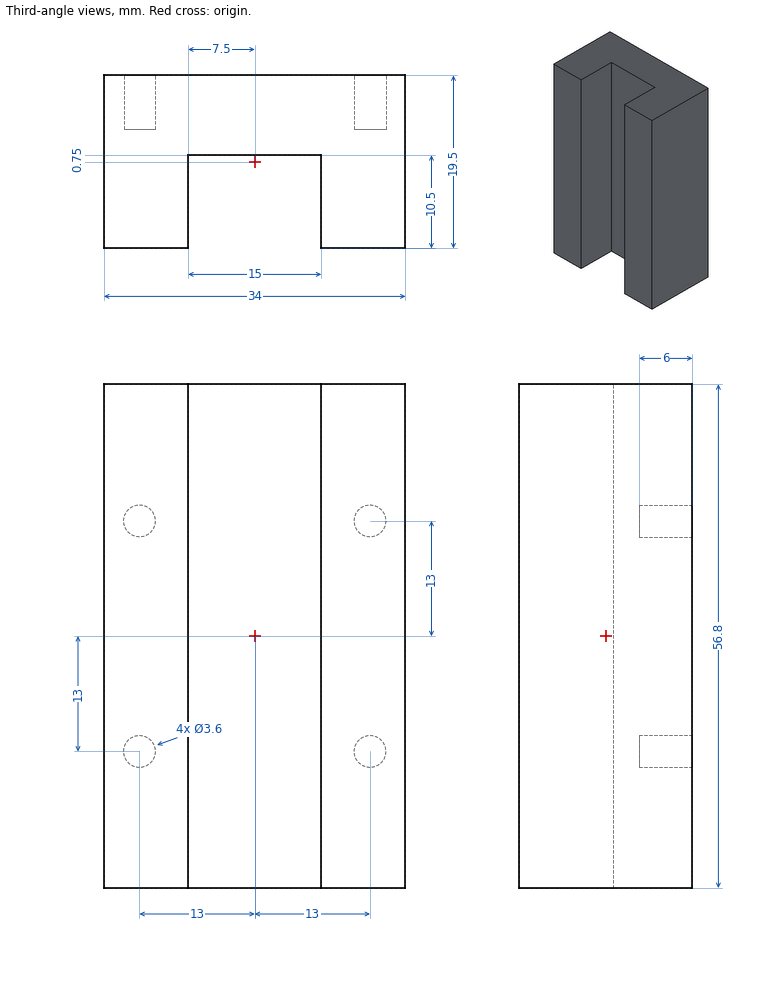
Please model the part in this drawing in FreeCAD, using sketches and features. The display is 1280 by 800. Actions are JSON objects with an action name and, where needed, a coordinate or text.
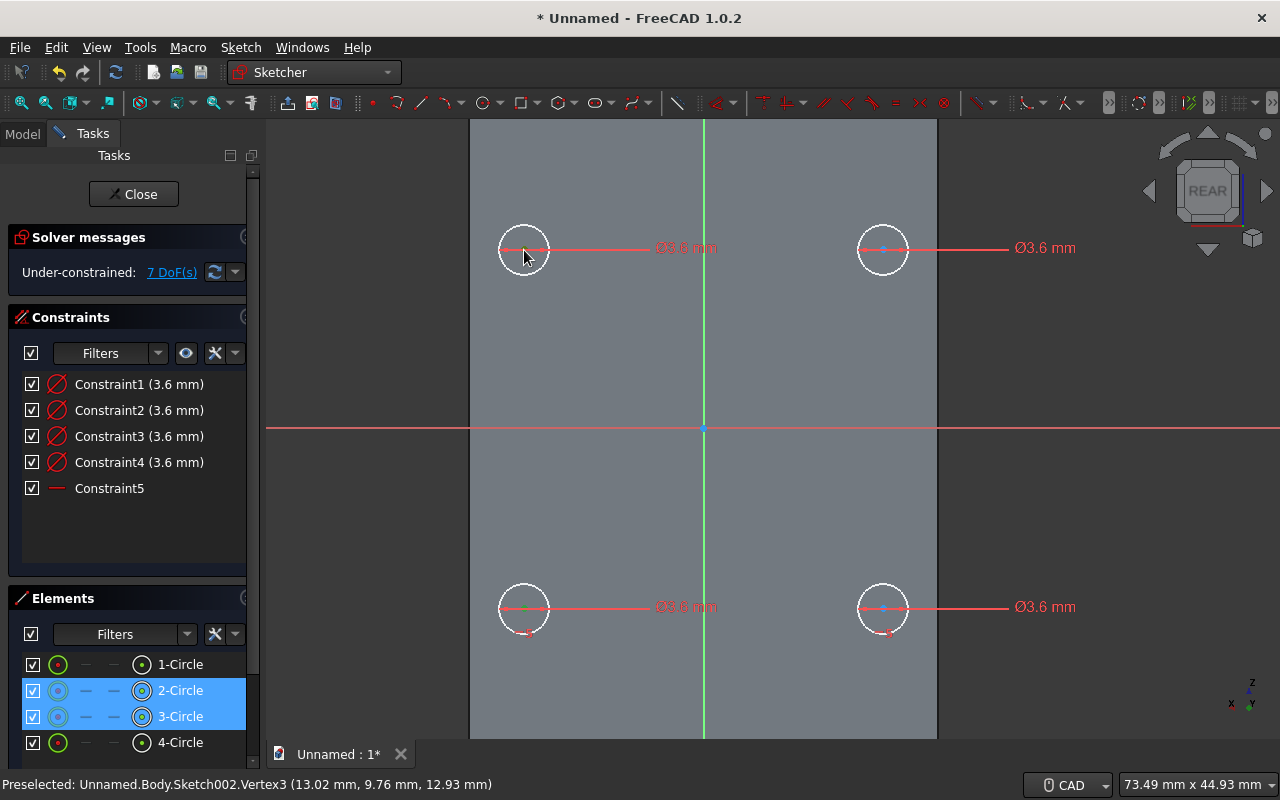
{"action": "key", "text": "v"}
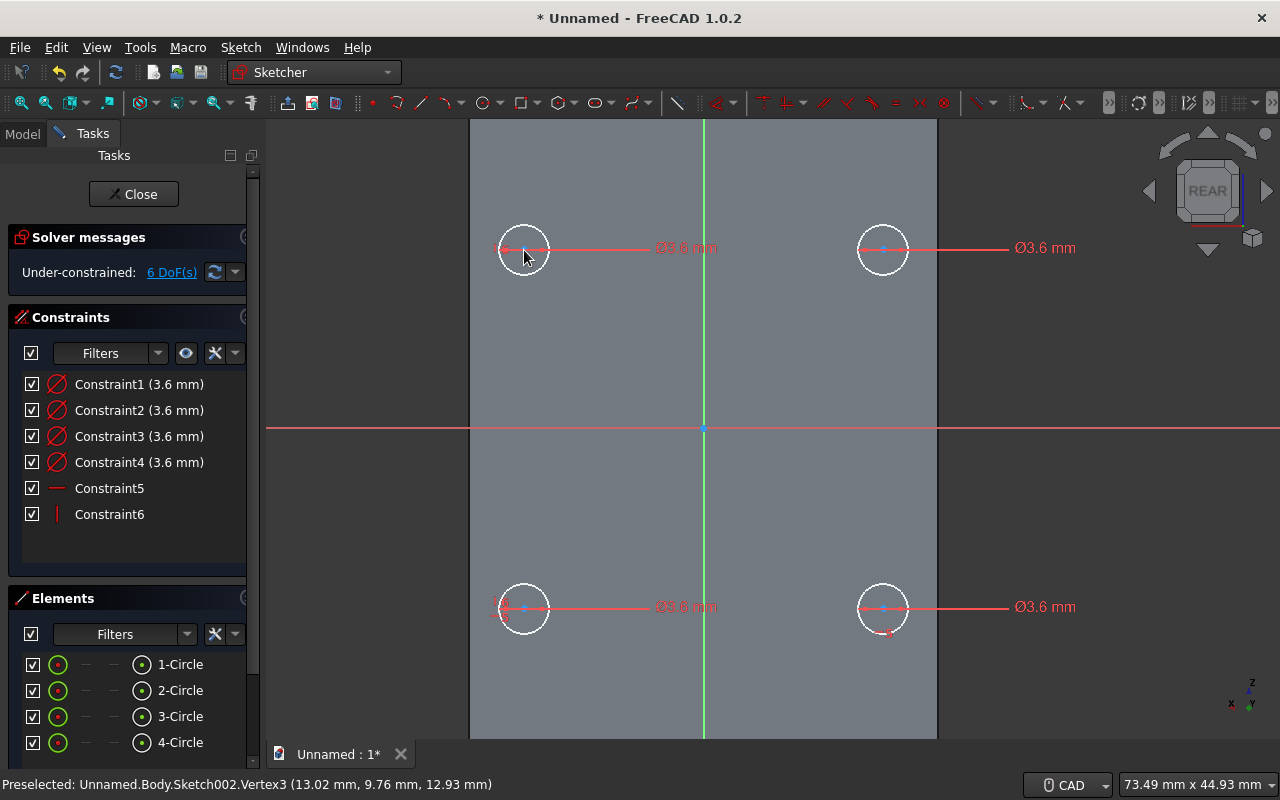
{"action": "left_click", "coordinate": [883, 609]}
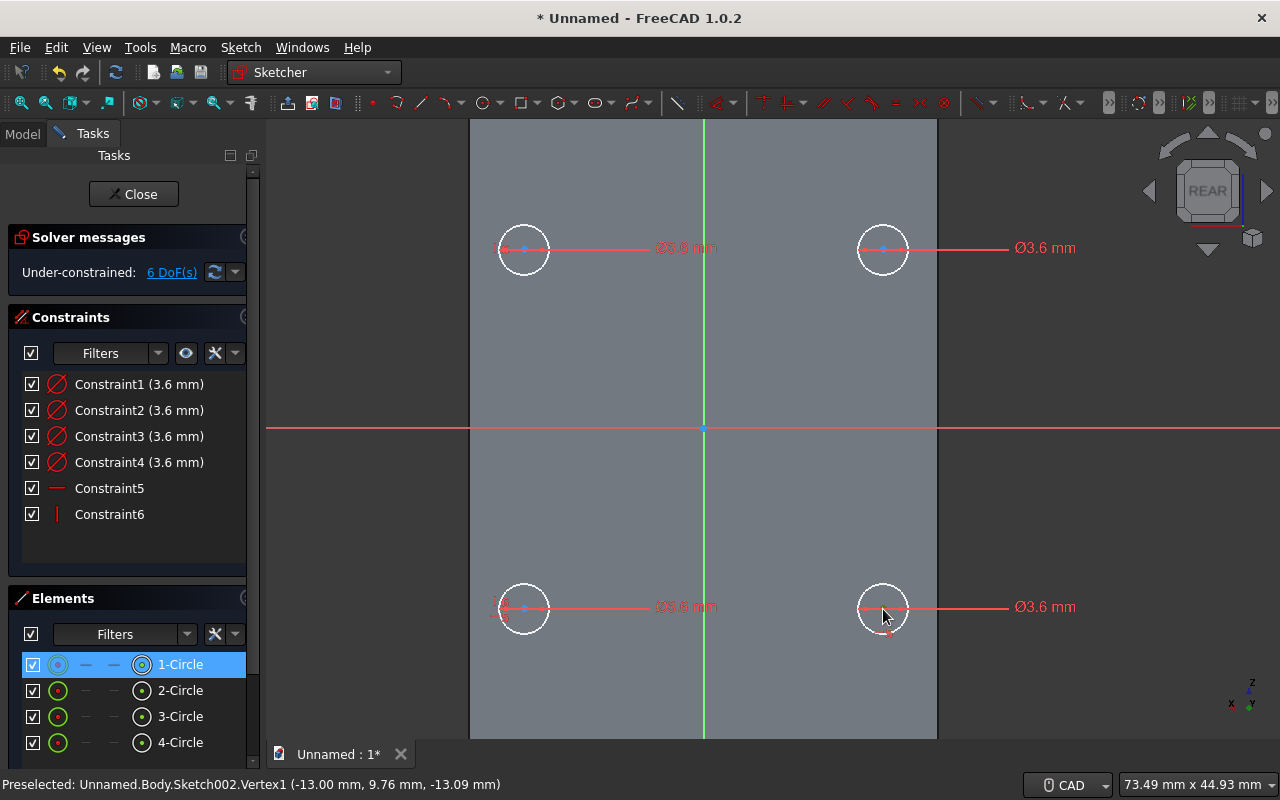
{"action": "left_click", "coordinate": [883, 250]}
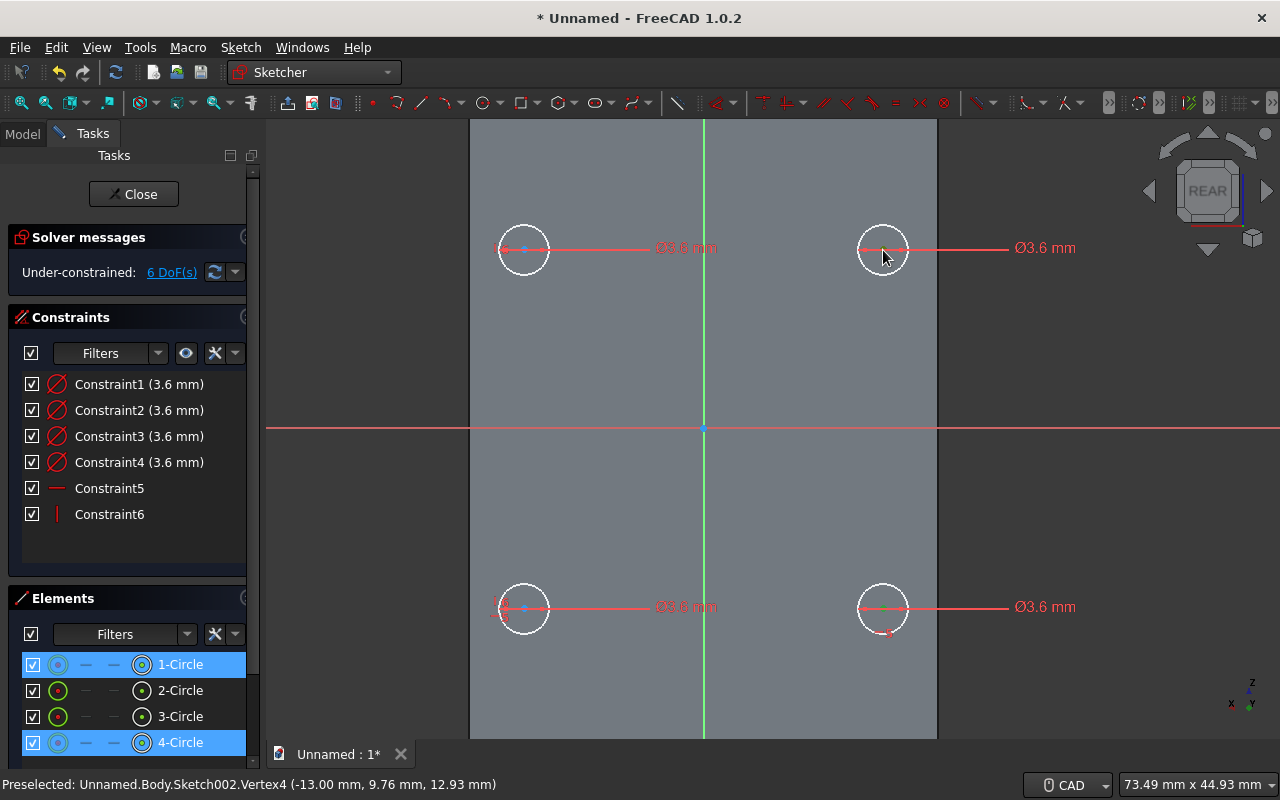
{"action": "key", "text": "v"}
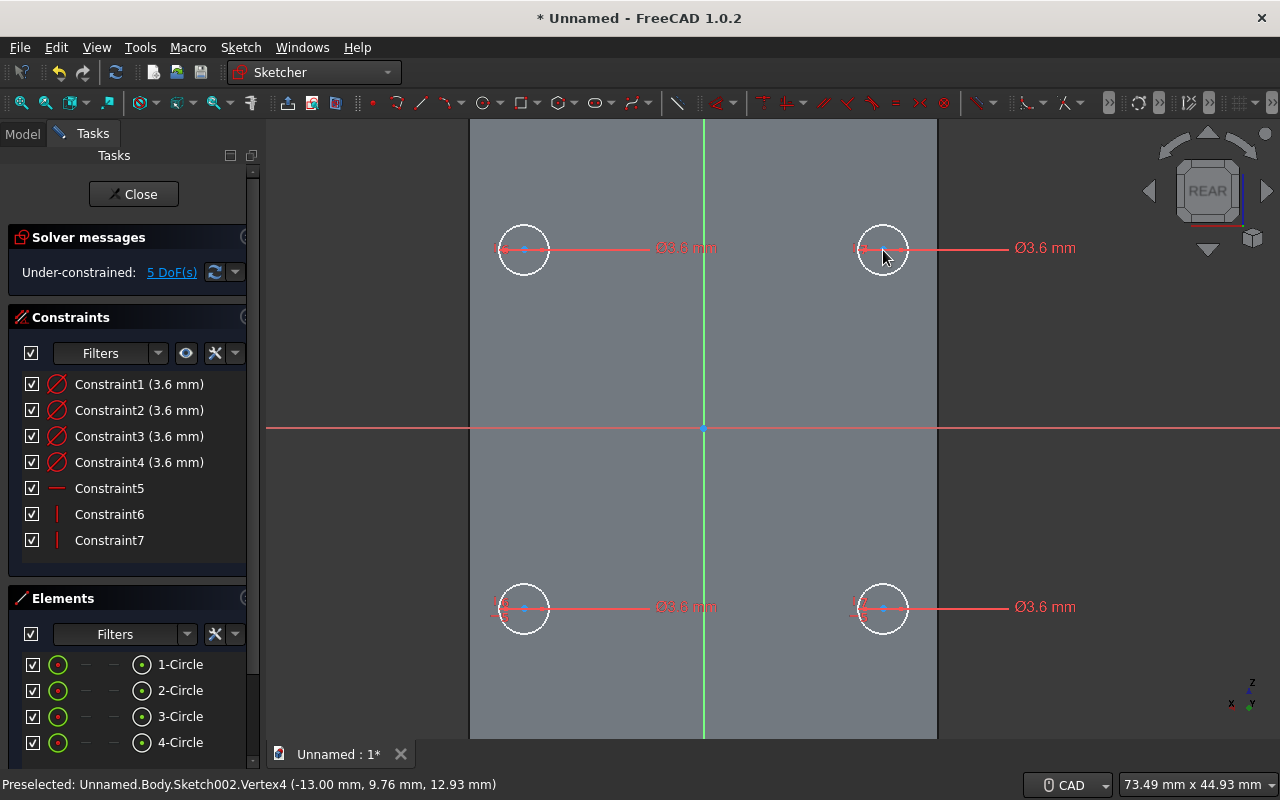
{"action": "left_click", "coordinate": [524, 250]}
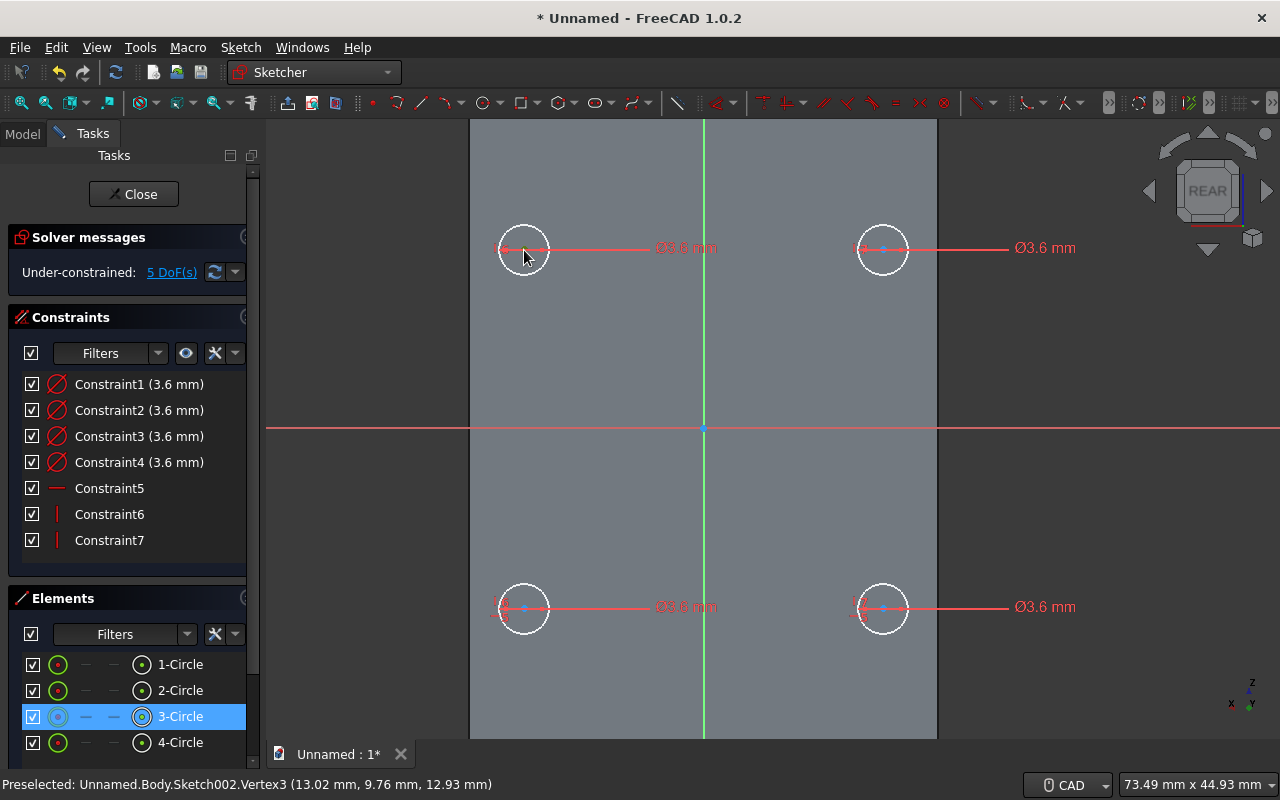
{"action": "left_click", "coordinate": [883, 250]}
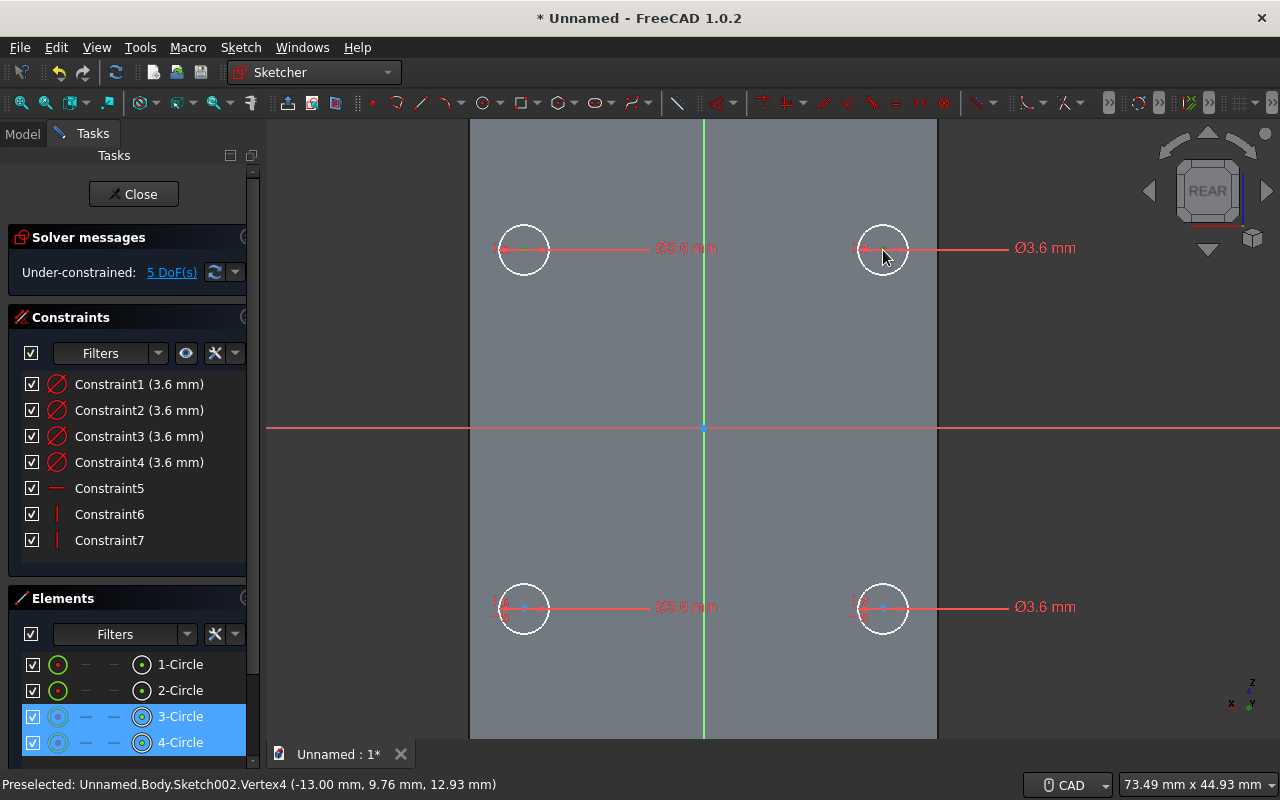
{"action": "left_click", "coordinate": [806, 104]}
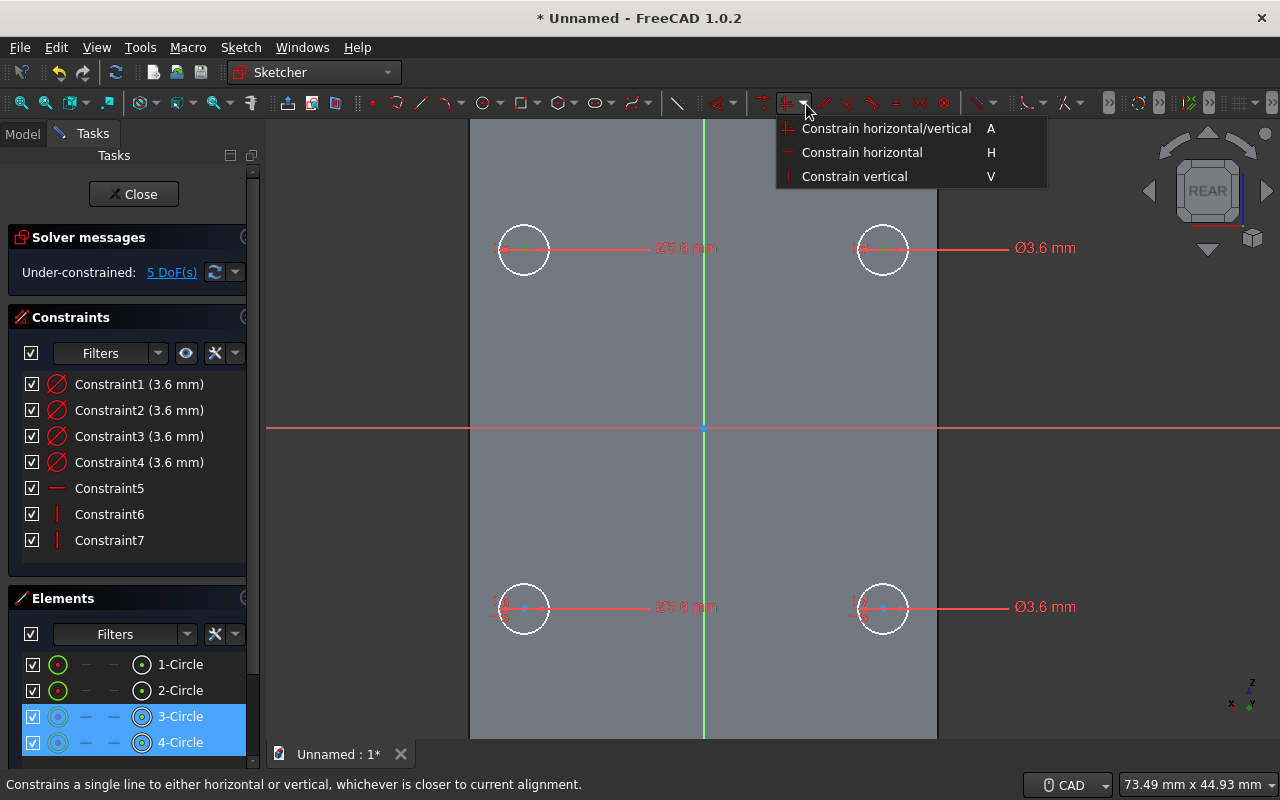
{"action": "left_click", "coordinate": [912, 152]}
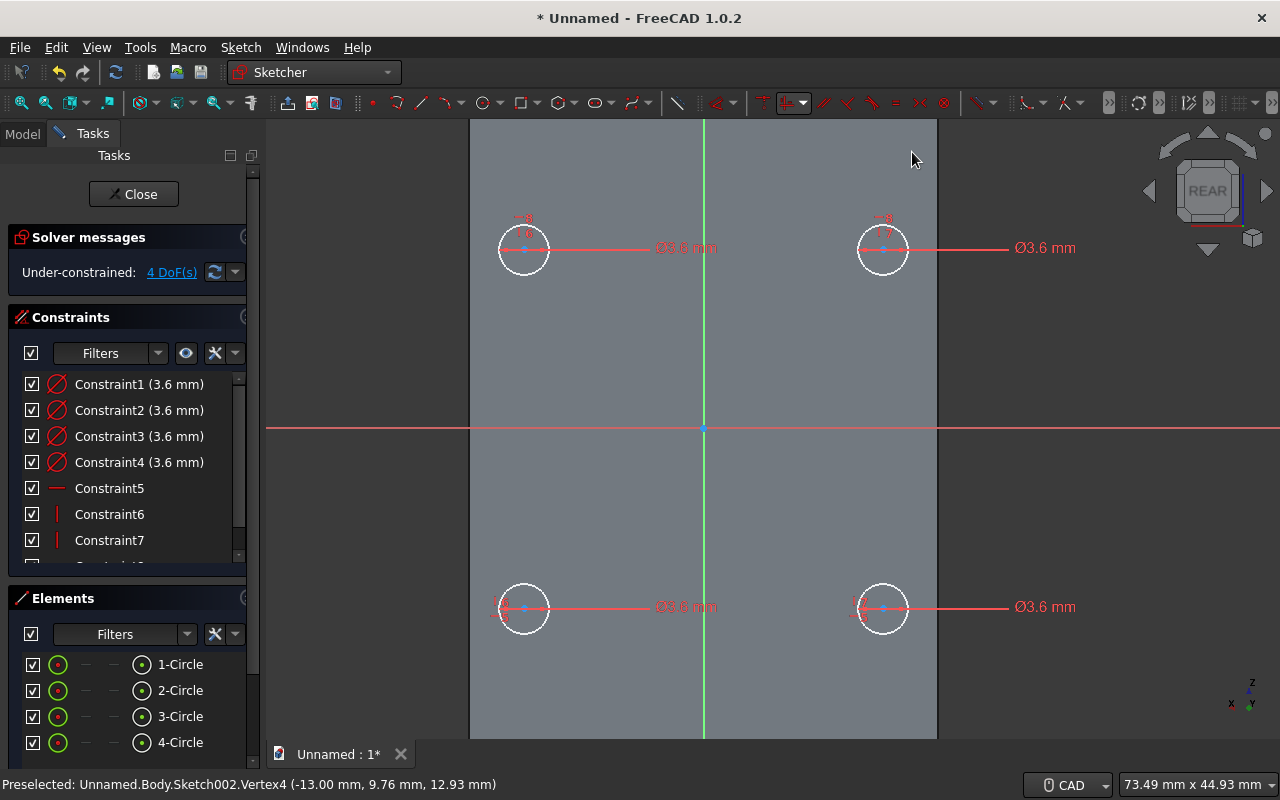
{"action": "left_click", "coordinate": [716, 104]}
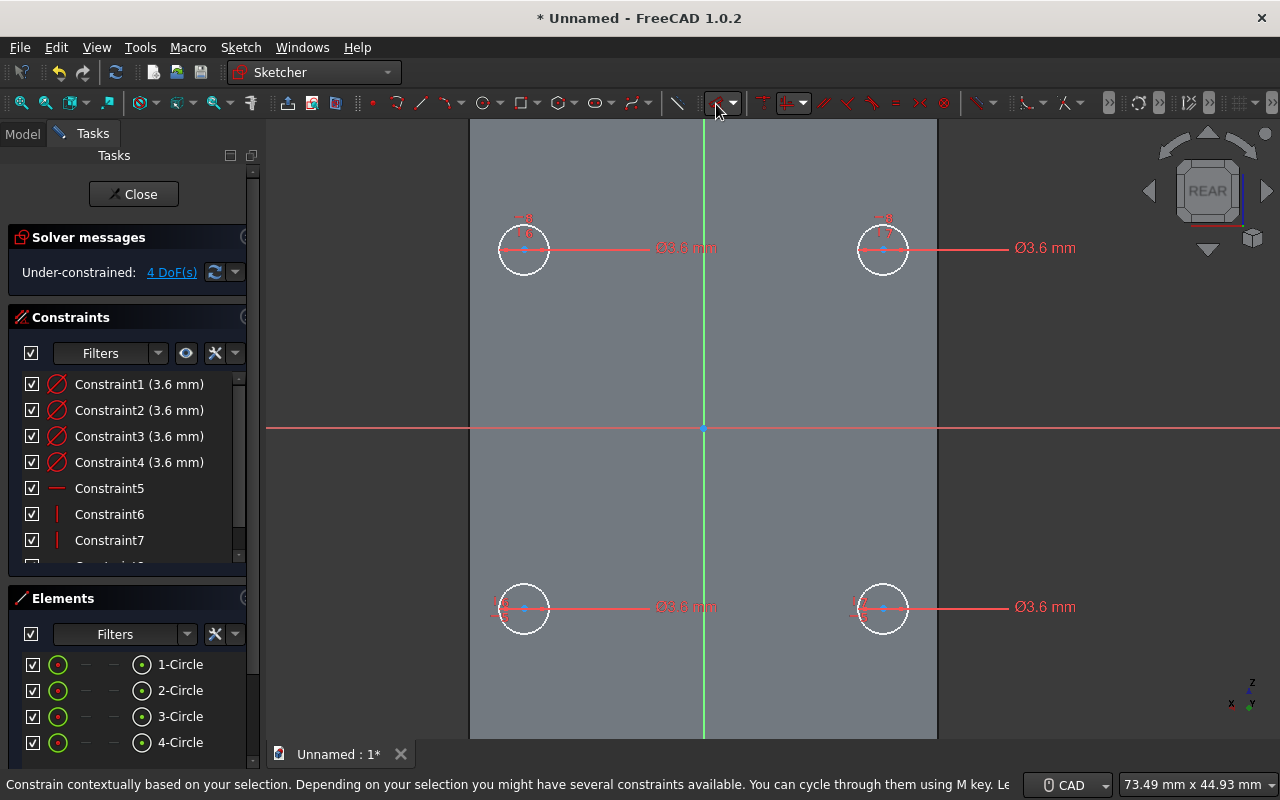
{"action": "left_click", "coordinate": [883, 609]}
{"action": "left_click", "coordinate": [793, 643]}